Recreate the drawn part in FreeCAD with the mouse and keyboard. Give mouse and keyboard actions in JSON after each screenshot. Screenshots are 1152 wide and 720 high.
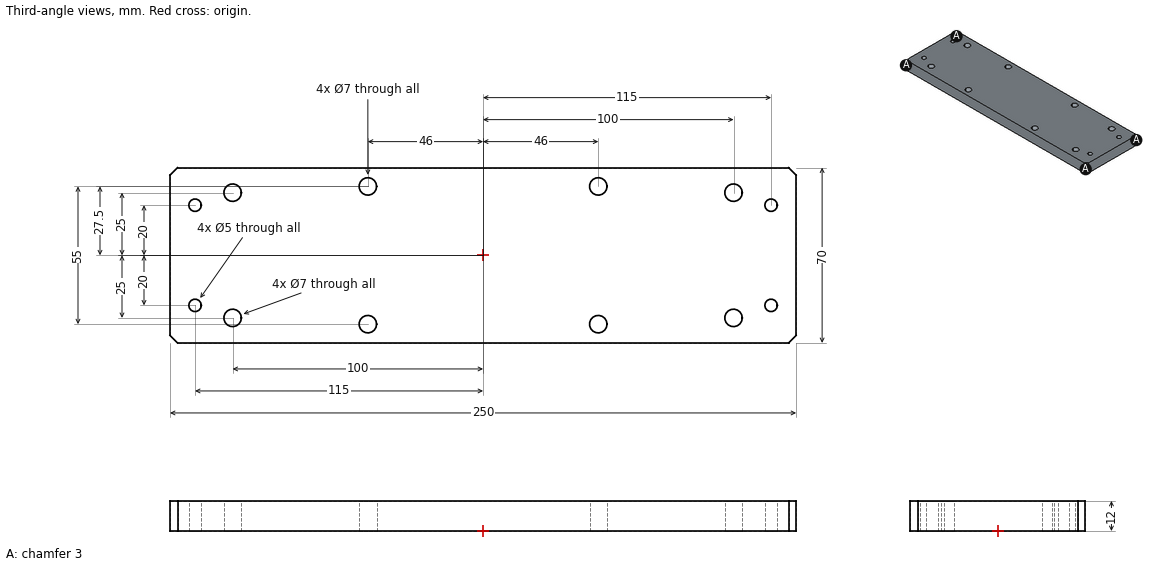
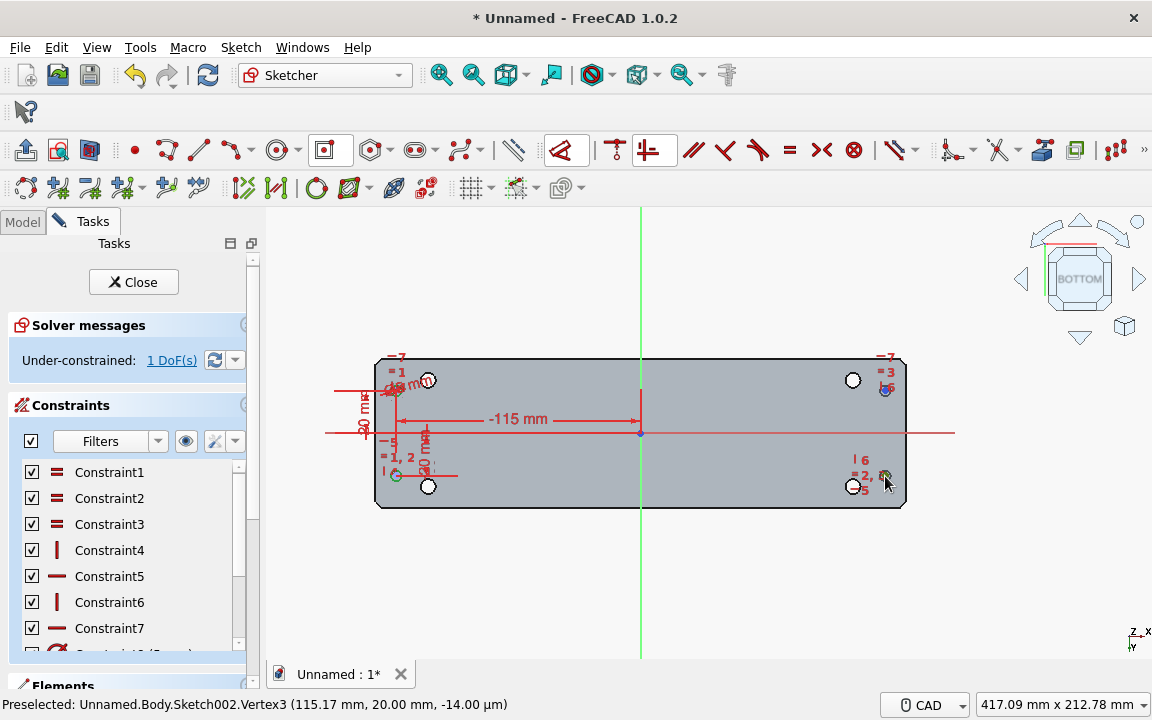
{"action": "left_click", "coordinate": [584, 150]}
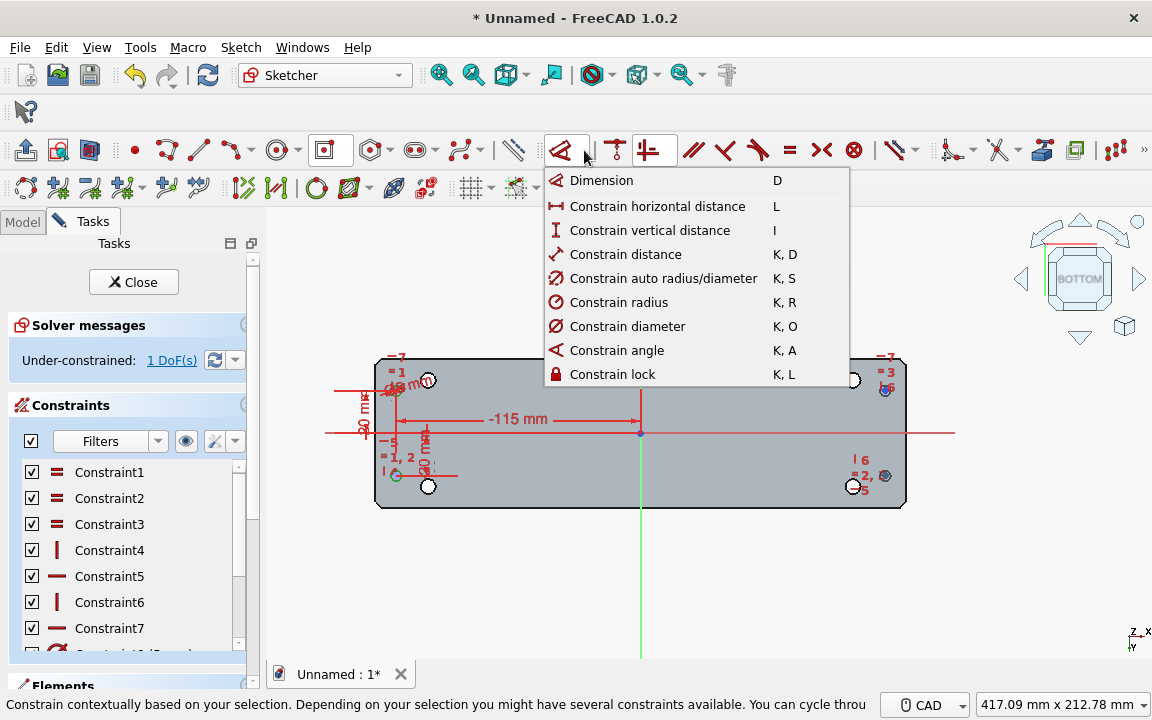
{"action": "left_click", "coordinate": [697, 206]}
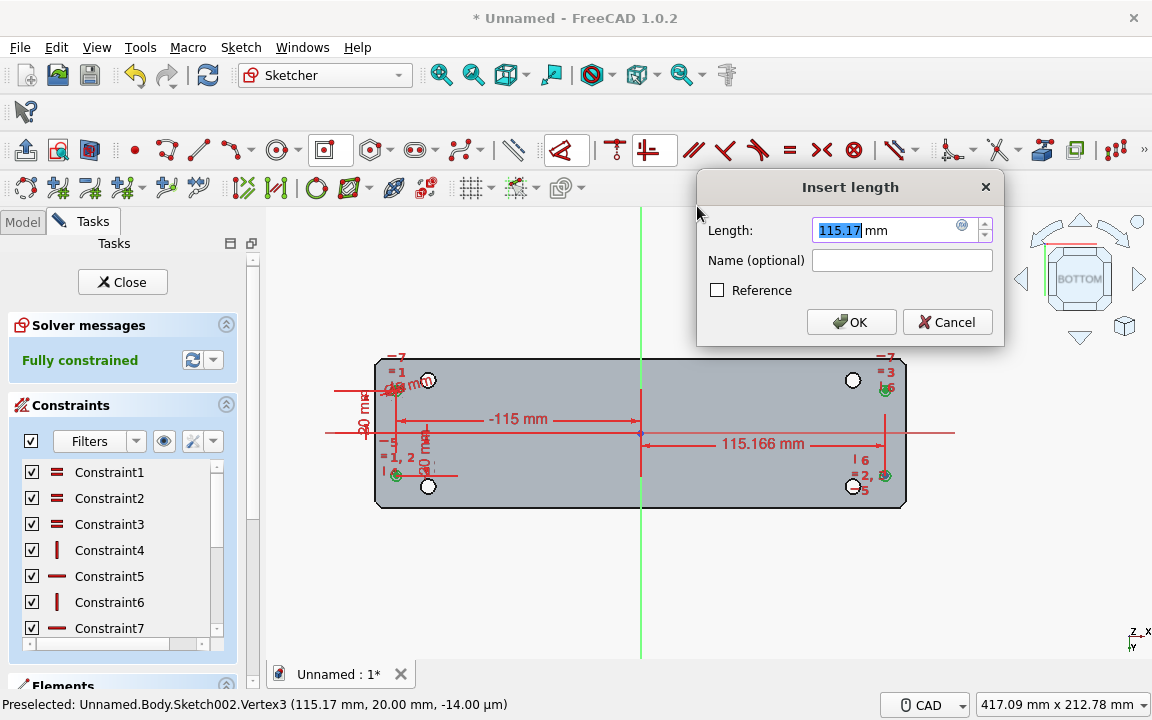
{"action": "type", "text": "115"}
{"action": "key", "text": "Return"}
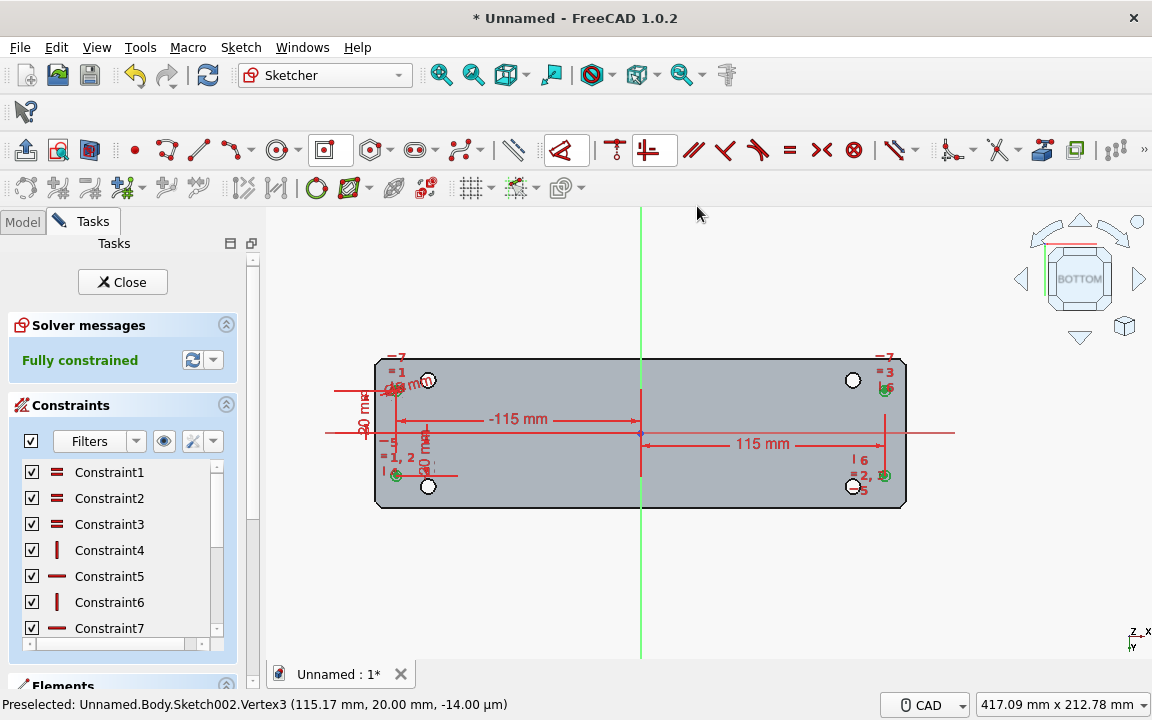
{"action": "left_click", "coordinate": [123, 282]}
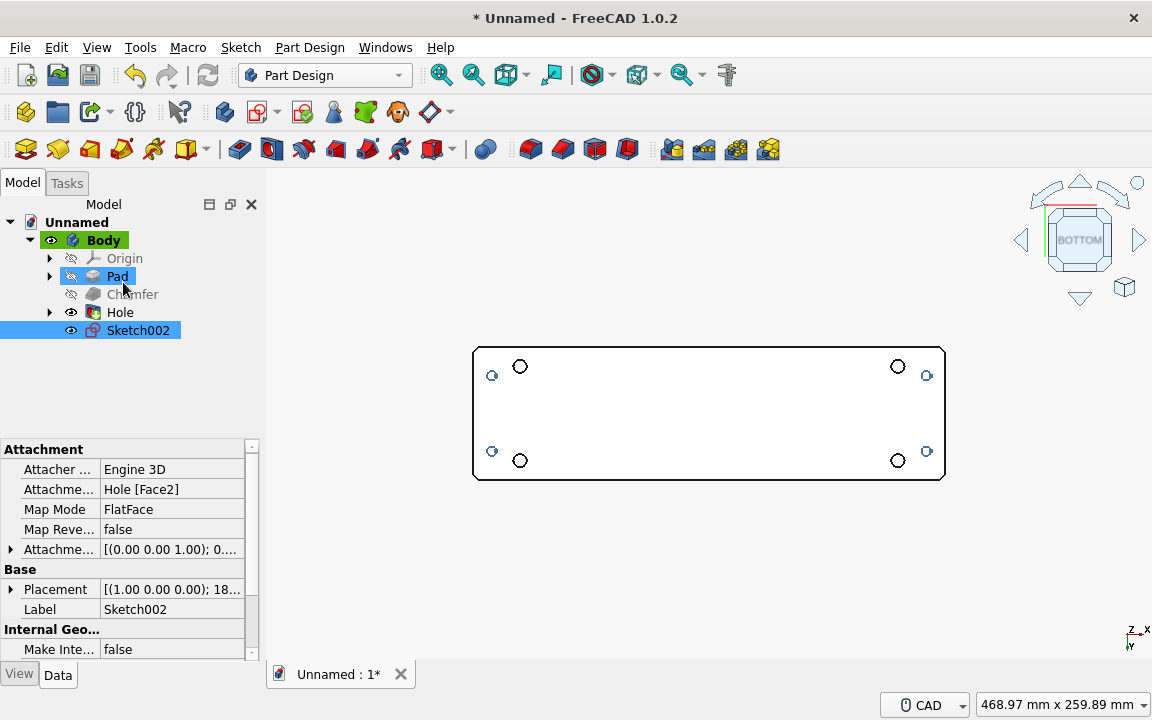
{"action": "left_click", "coordinate": [272, 150]}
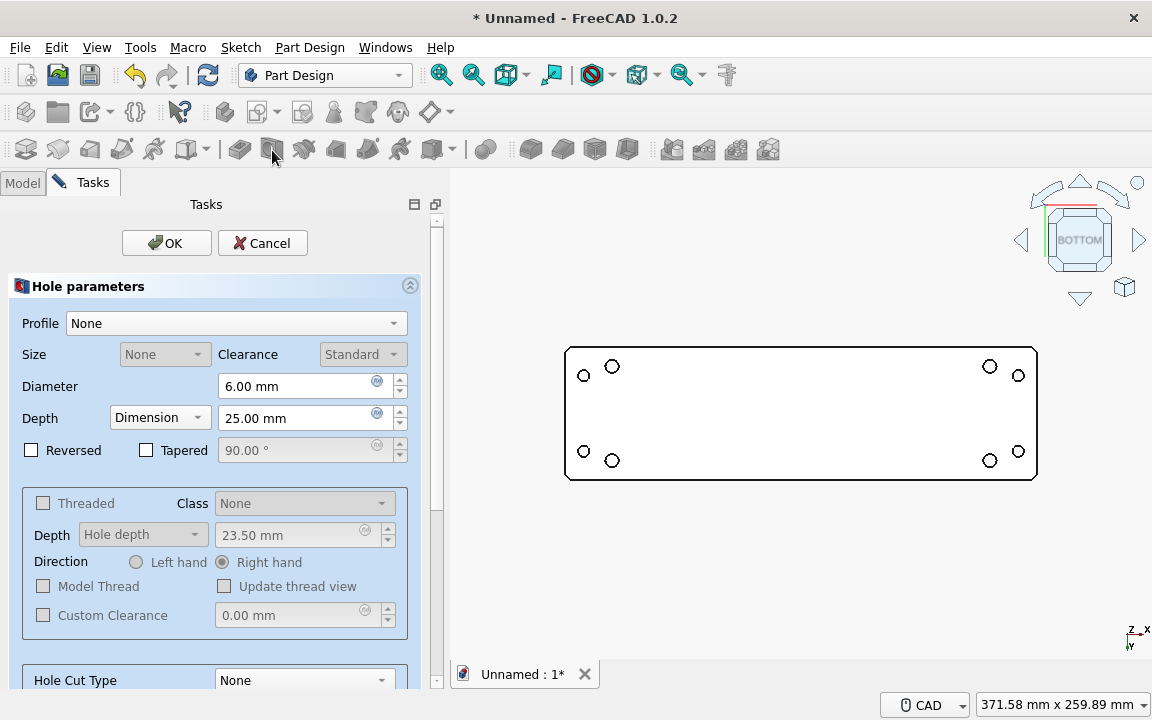
{"action": "triple_click", "coordinate": [305, 386]}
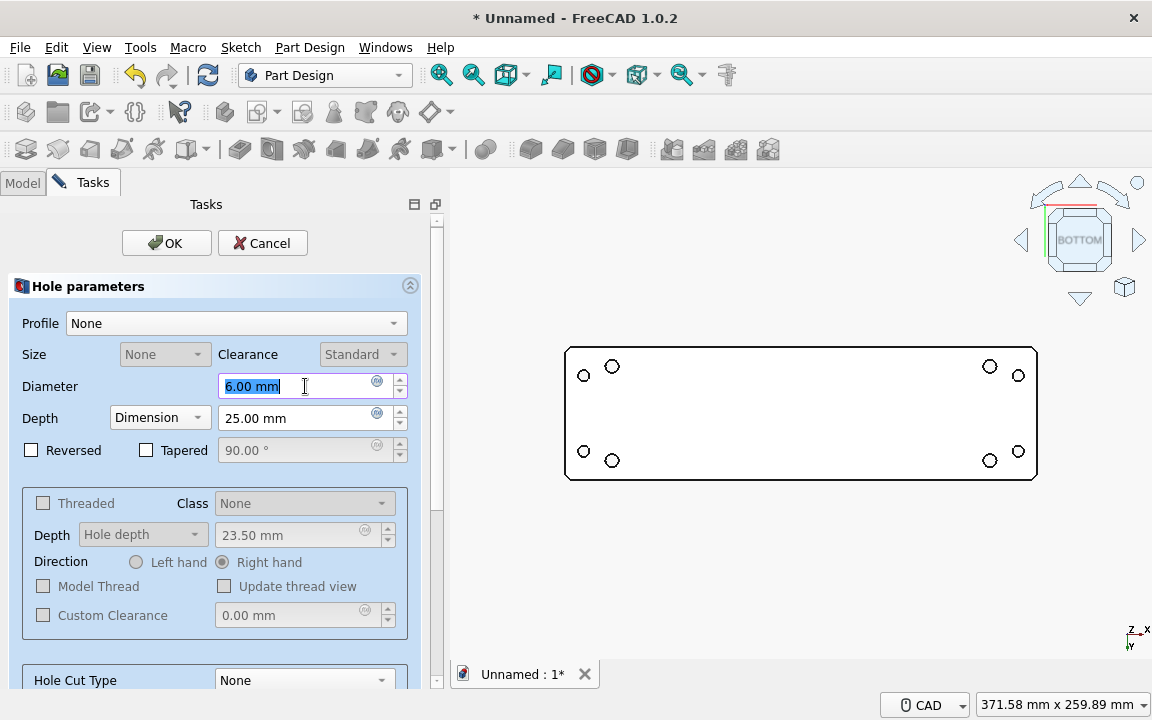
{"action": "type", "text": "5"}
{"action": "key", "text": "Tab"}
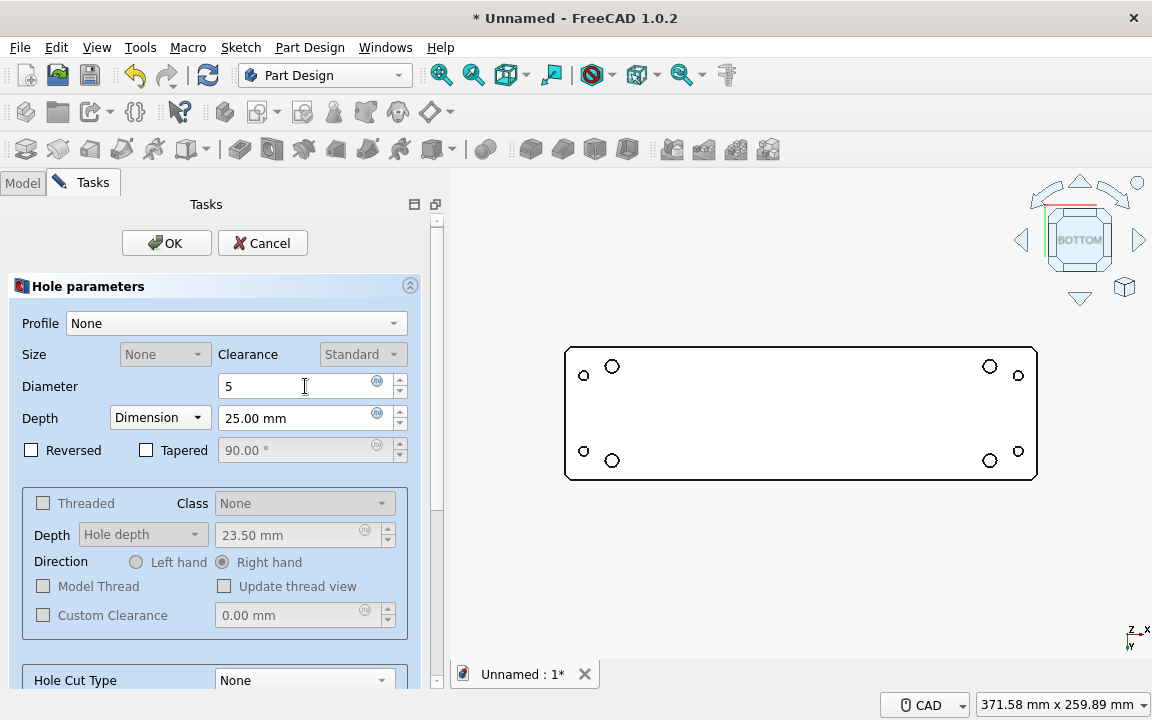
{"action": "left_click", "coordinate": [161, 418]}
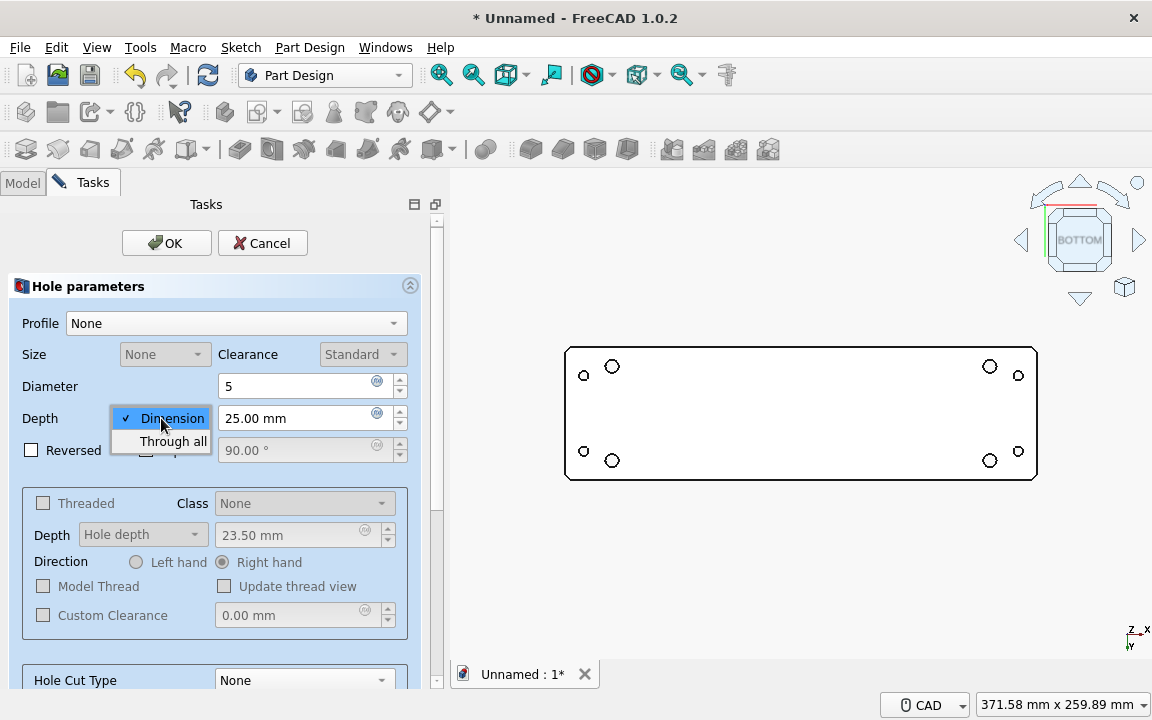
{"action": "left_click", "coordinate": [160, 442]}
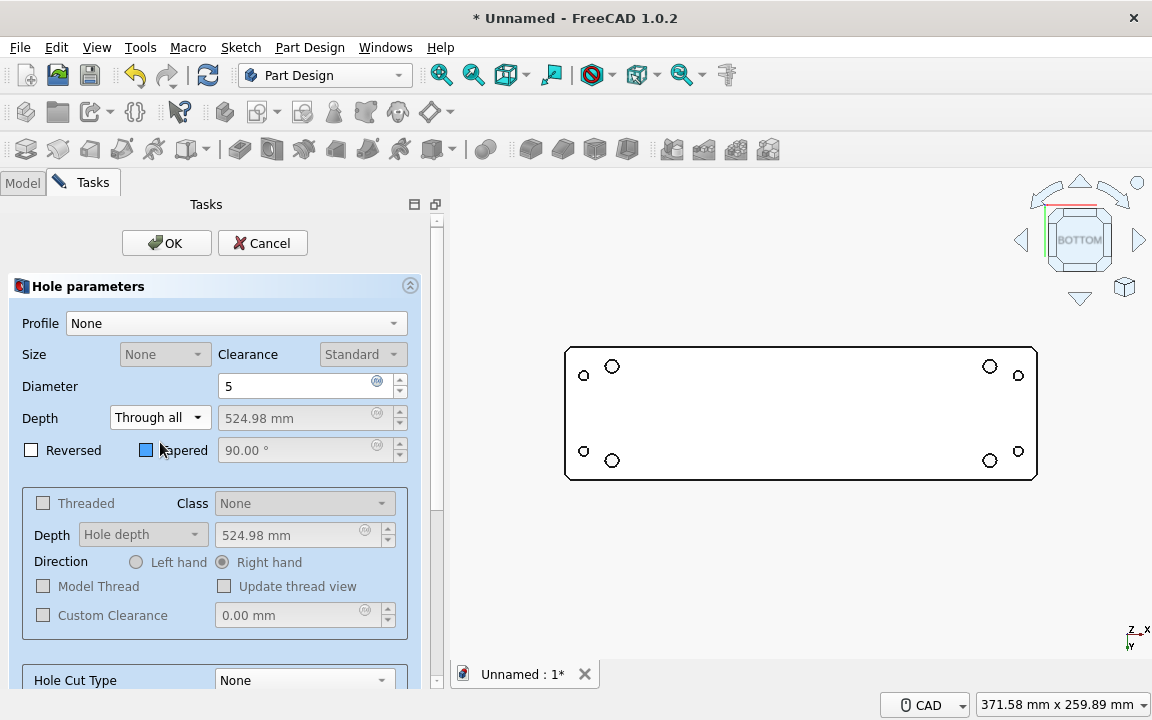
{"action": "left_click", "coordinate": [167, 243]}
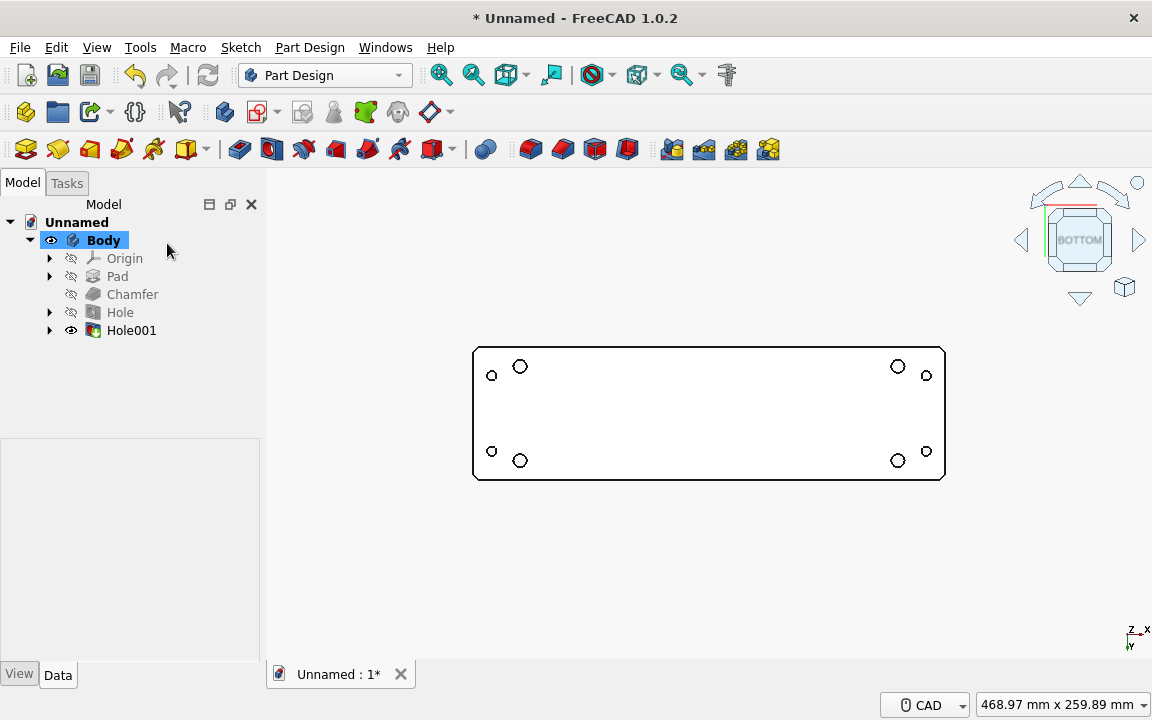
{"action": "left_click", "coordinate": [258, 112]}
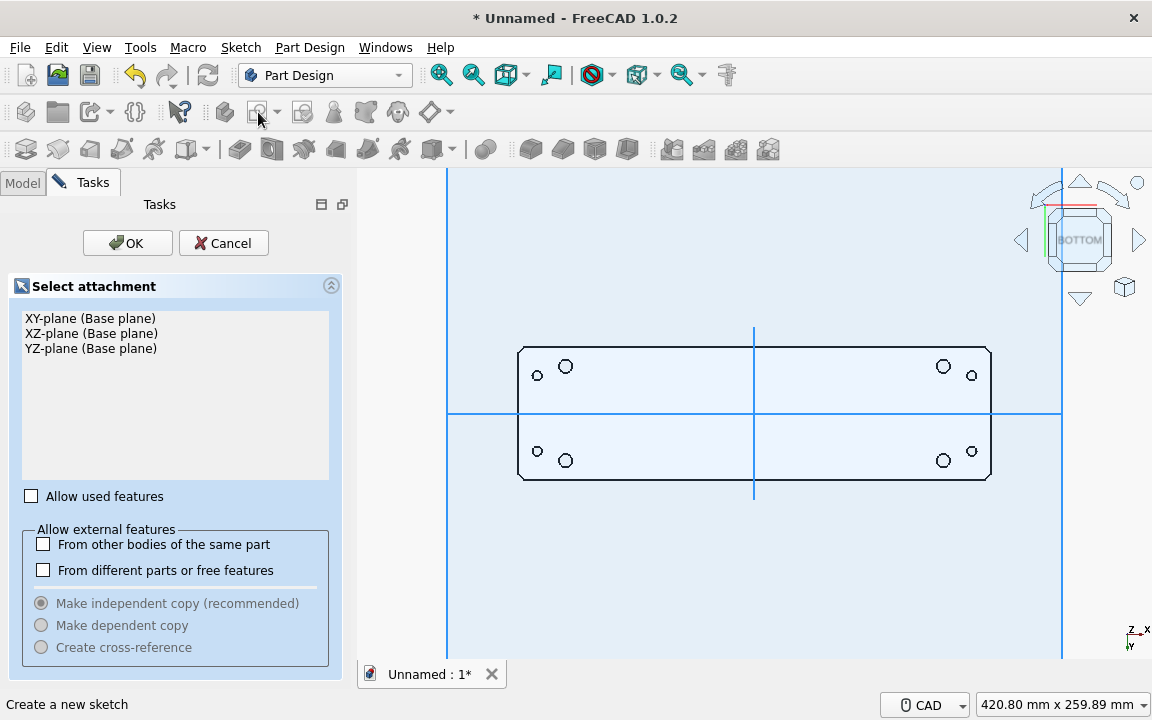
{"action": "left_click", "coordinate": [82, 318]}